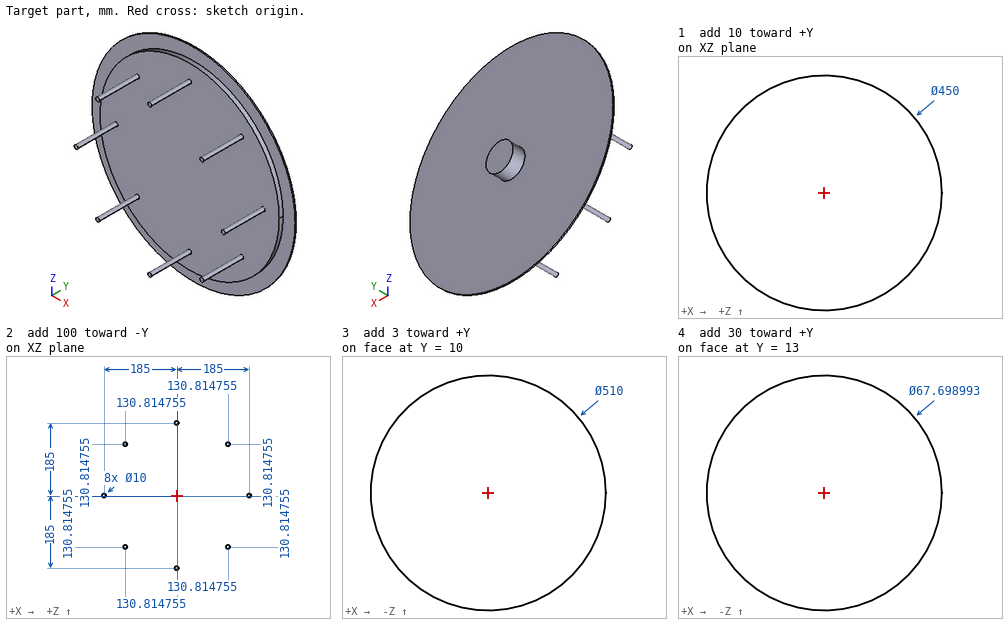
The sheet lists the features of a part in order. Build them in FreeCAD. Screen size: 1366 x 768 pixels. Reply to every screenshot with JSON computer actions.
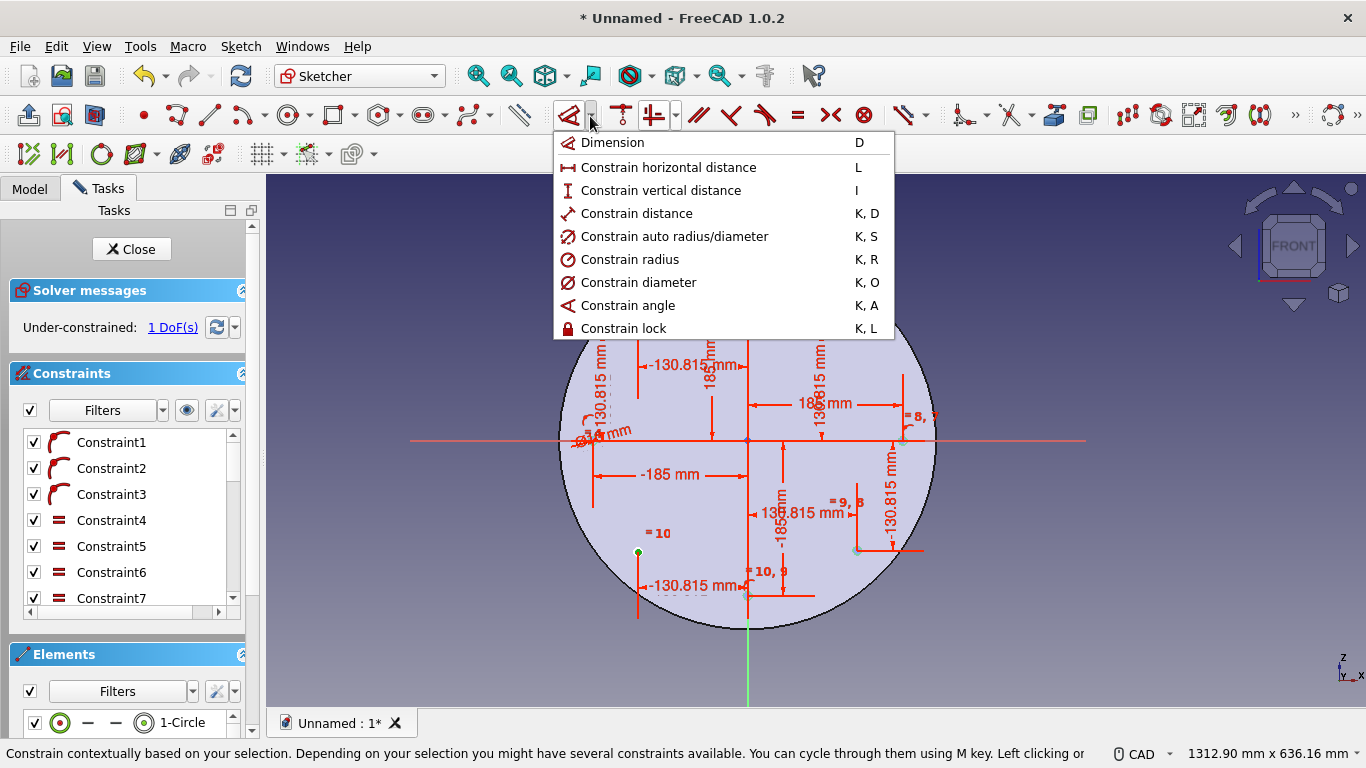
{"action": "left_click", "coordinate": [724, 190]}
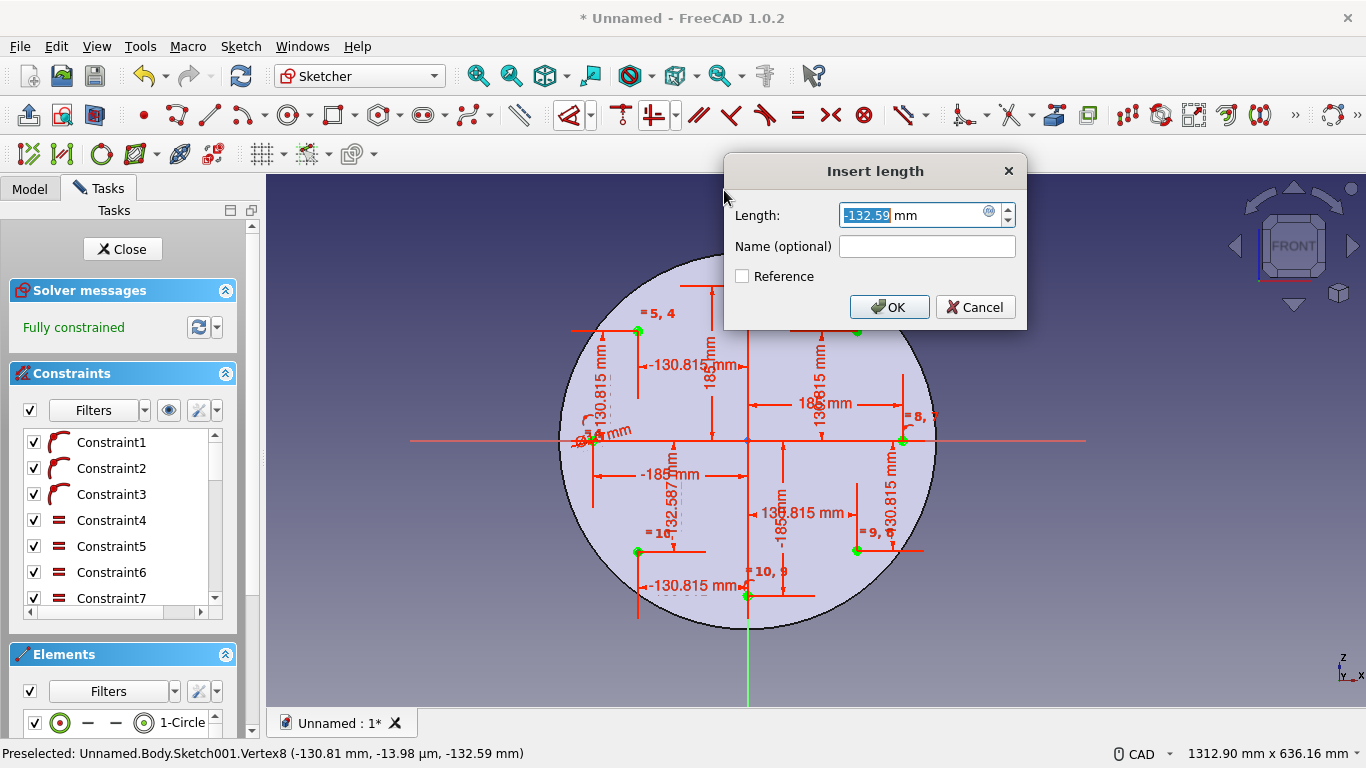
{"action": "type", "text": "-130.814755"}
{"action": "key", "text": "Return"}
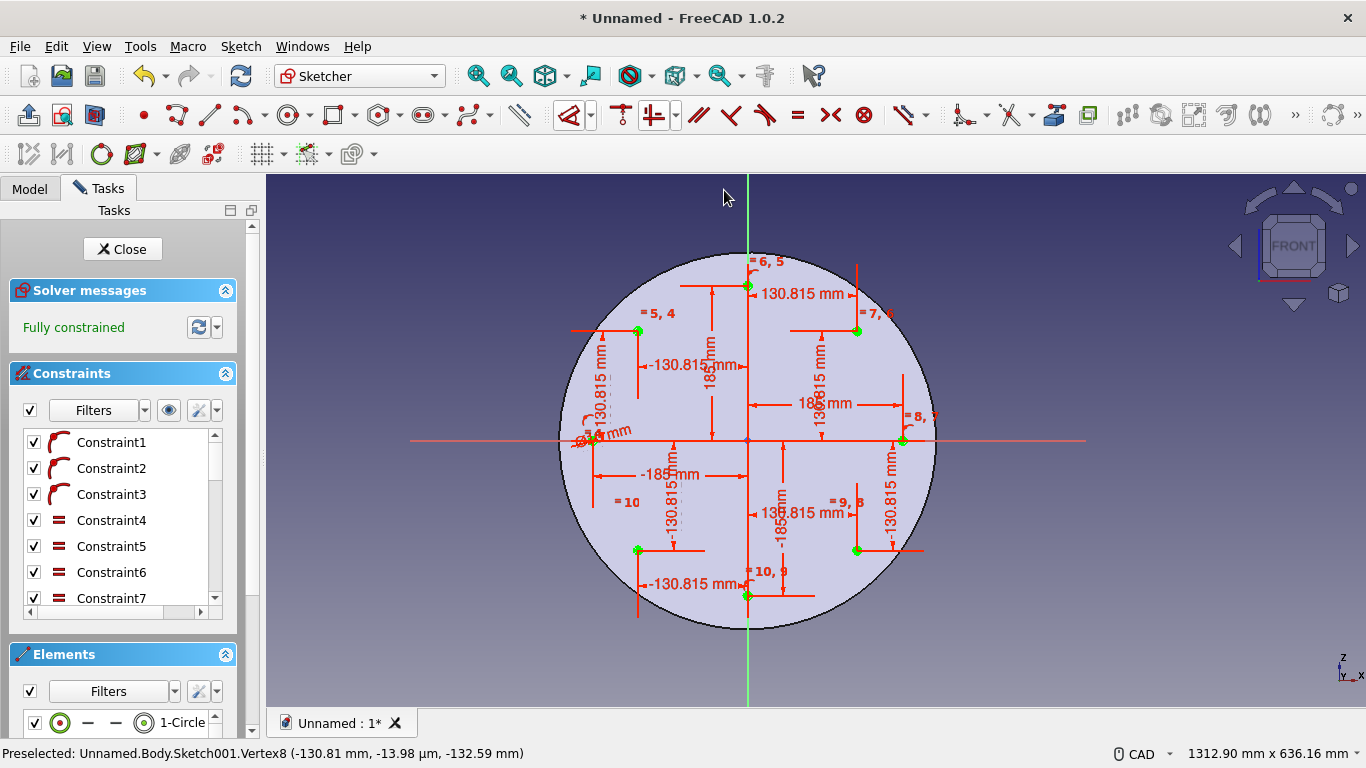
{"action": "left_click", "coordinate": [123, 249]}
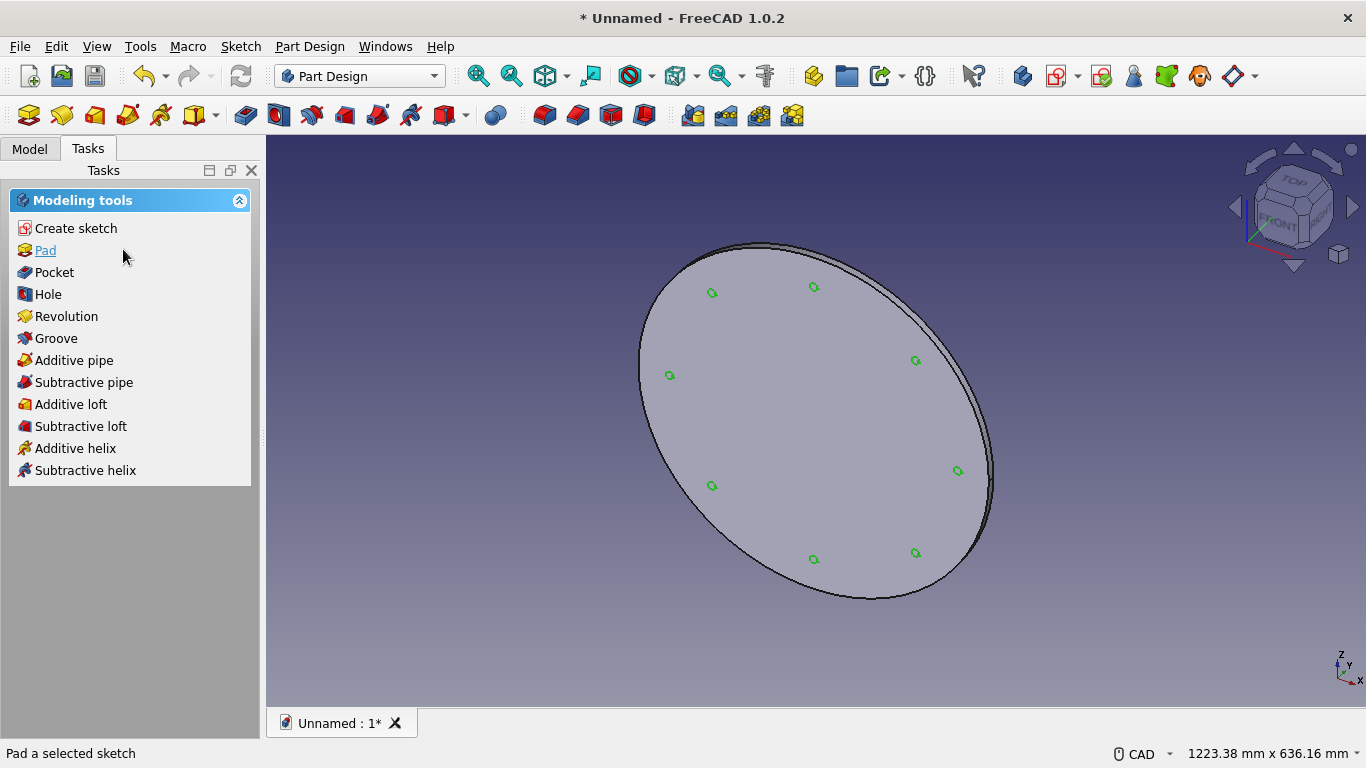
{"action": "left_click", "coordinate": [29, 116]}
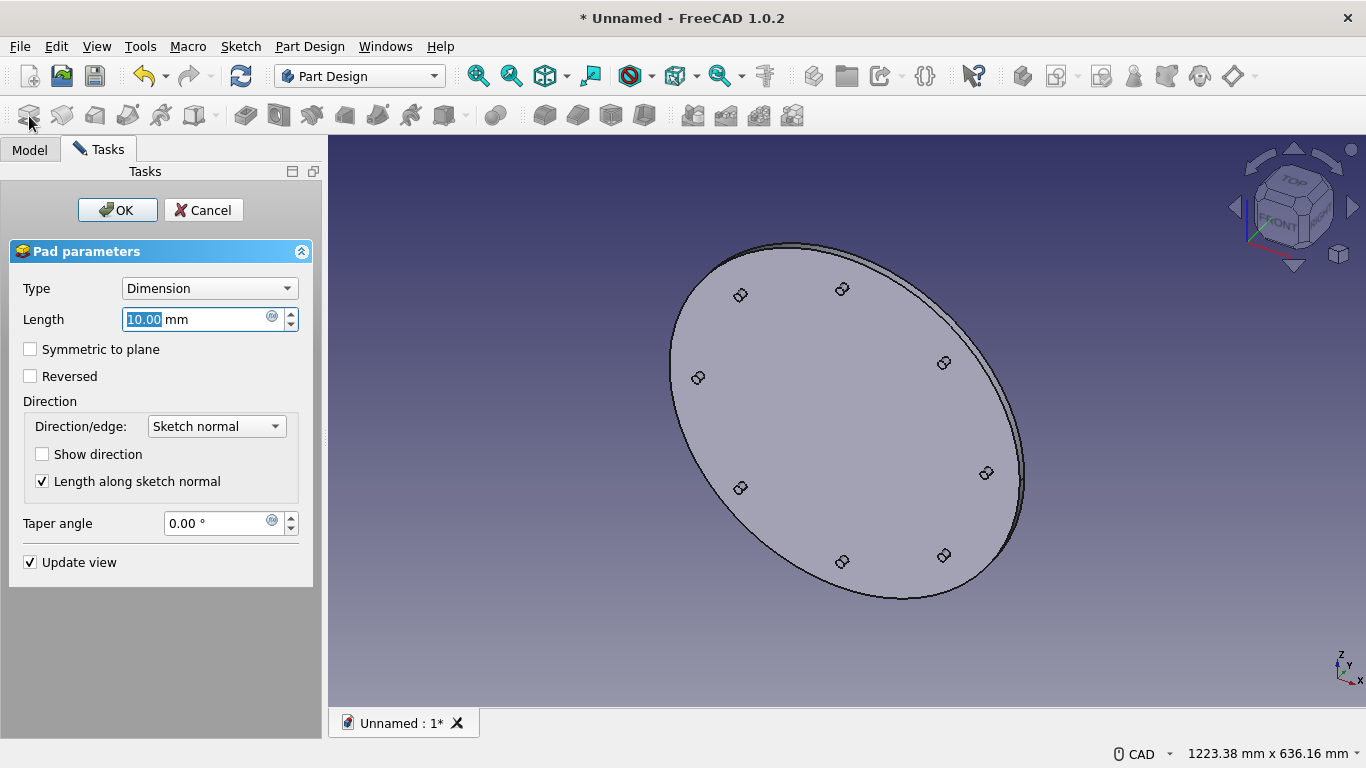
{"action": "type", "text": "100"}
{"action": "key", "text": "Tab"}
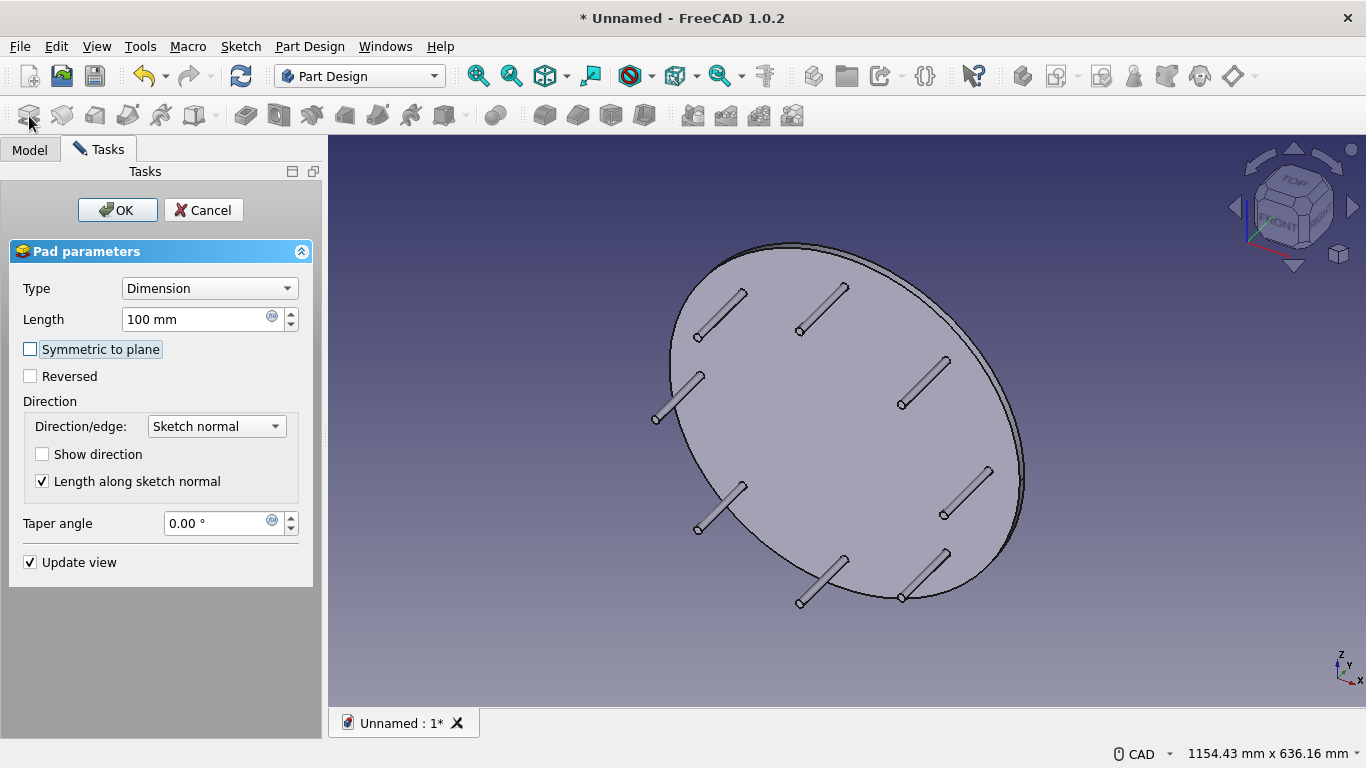
{"action": "left_click", "coordinate": [118, 210]}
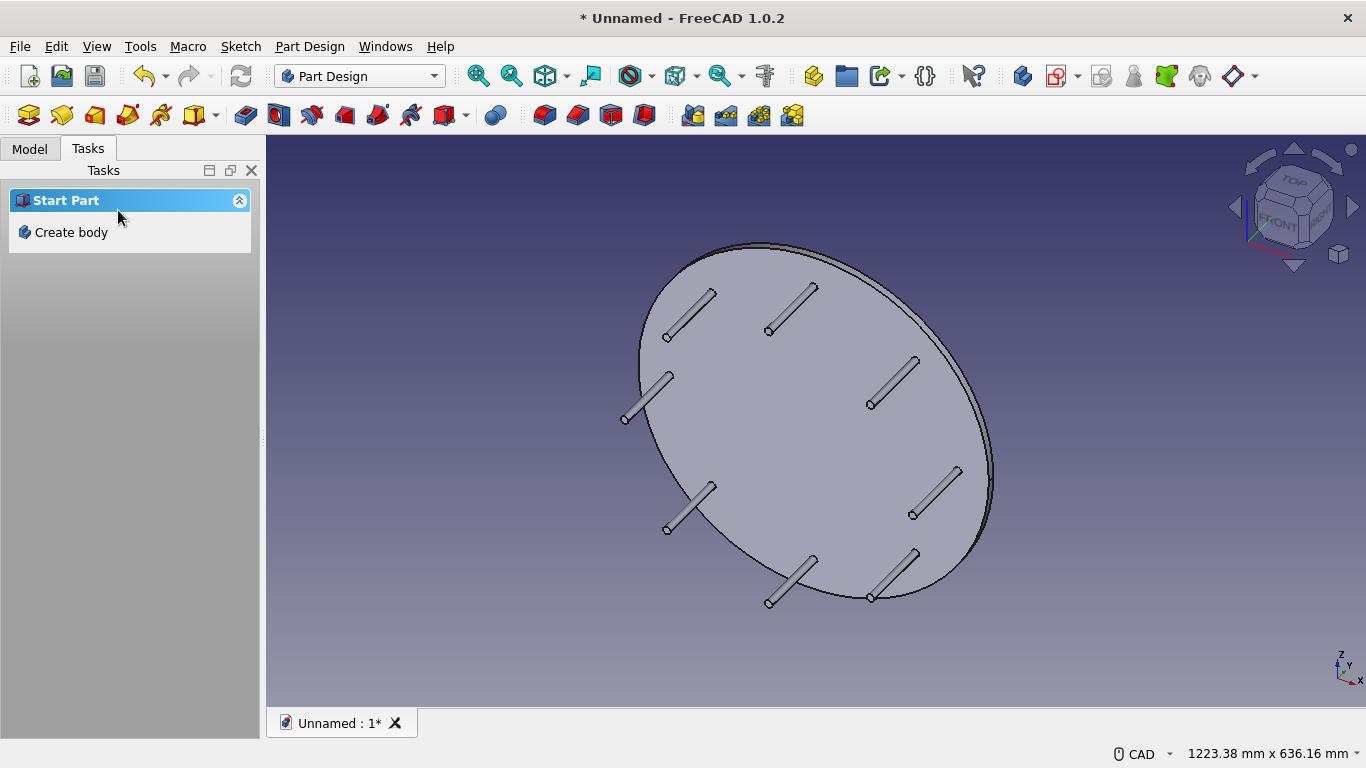
{"action": "key", "text": "4"}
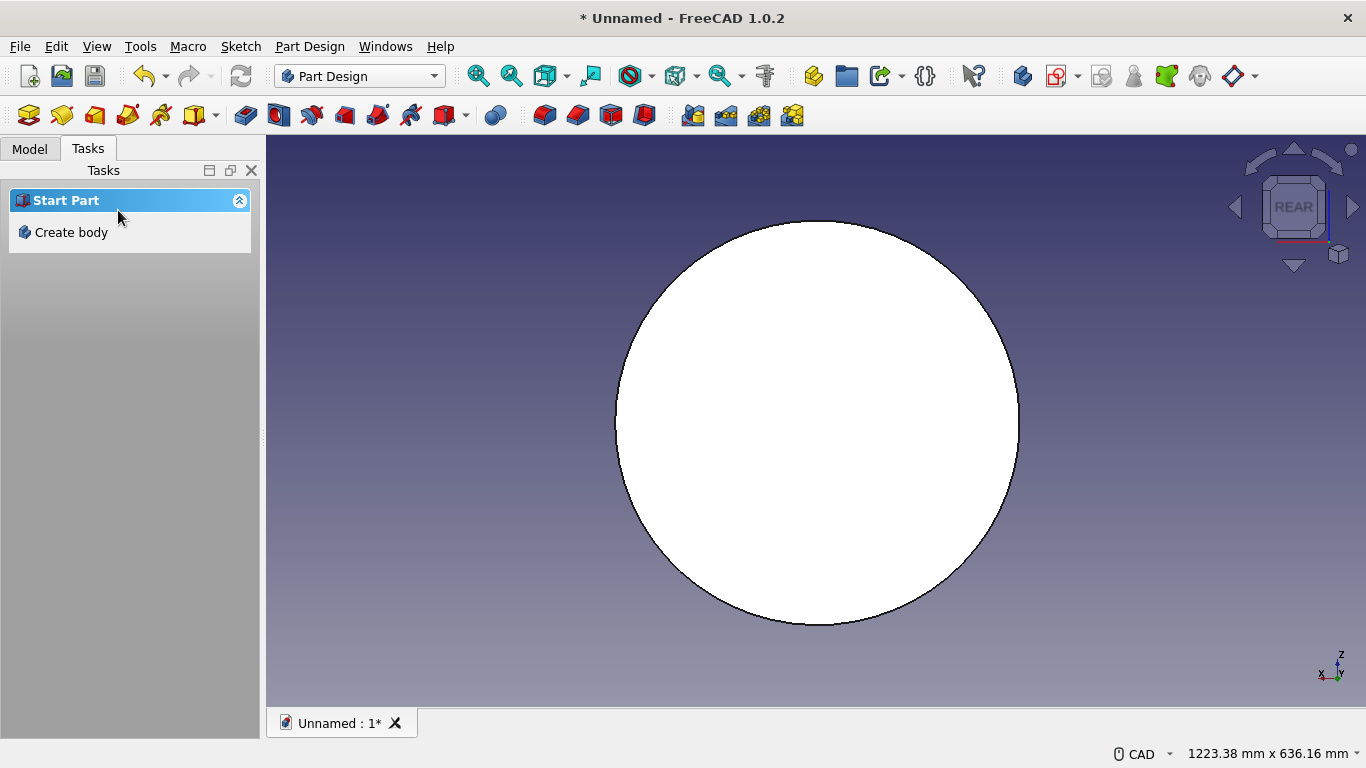
{"action": "left_click", "coordinate": [817, 422]}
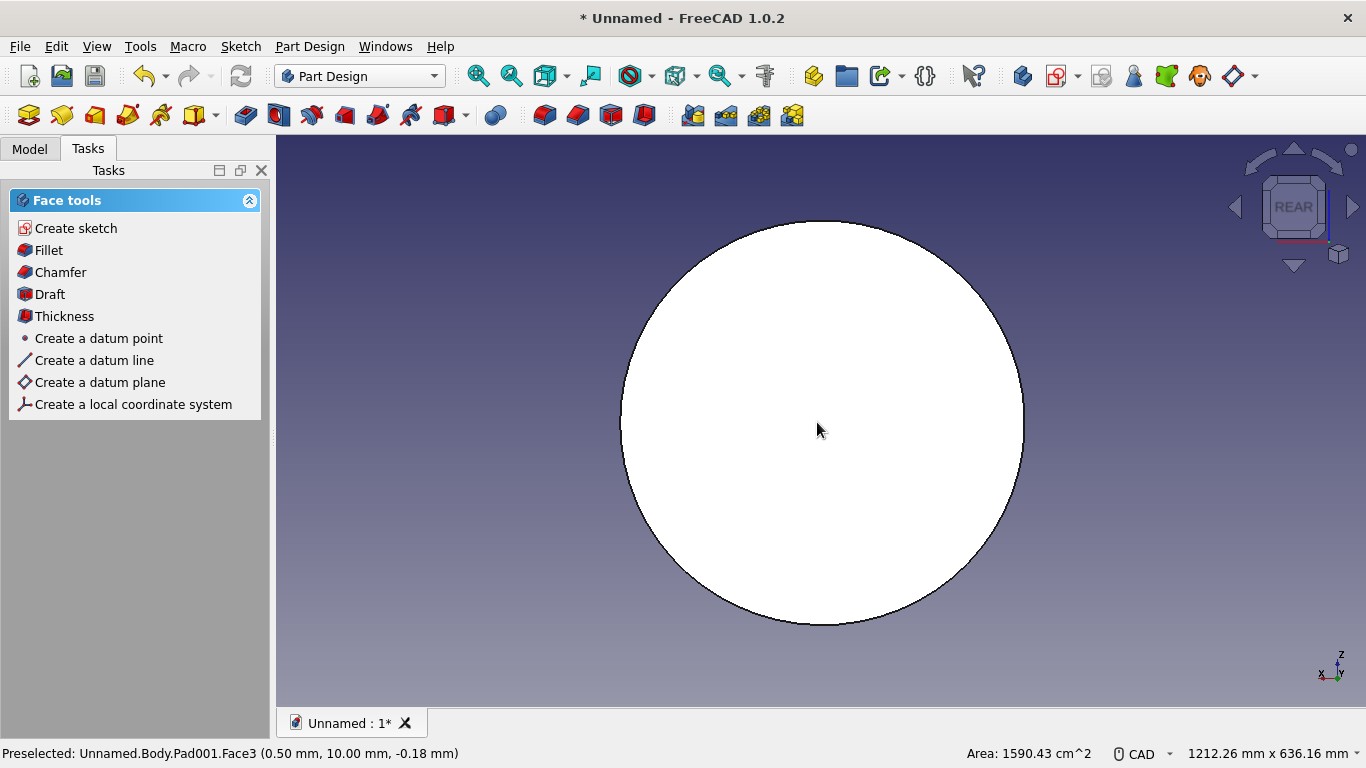
{"action": "left_click", "coordinate": [1056, 76]}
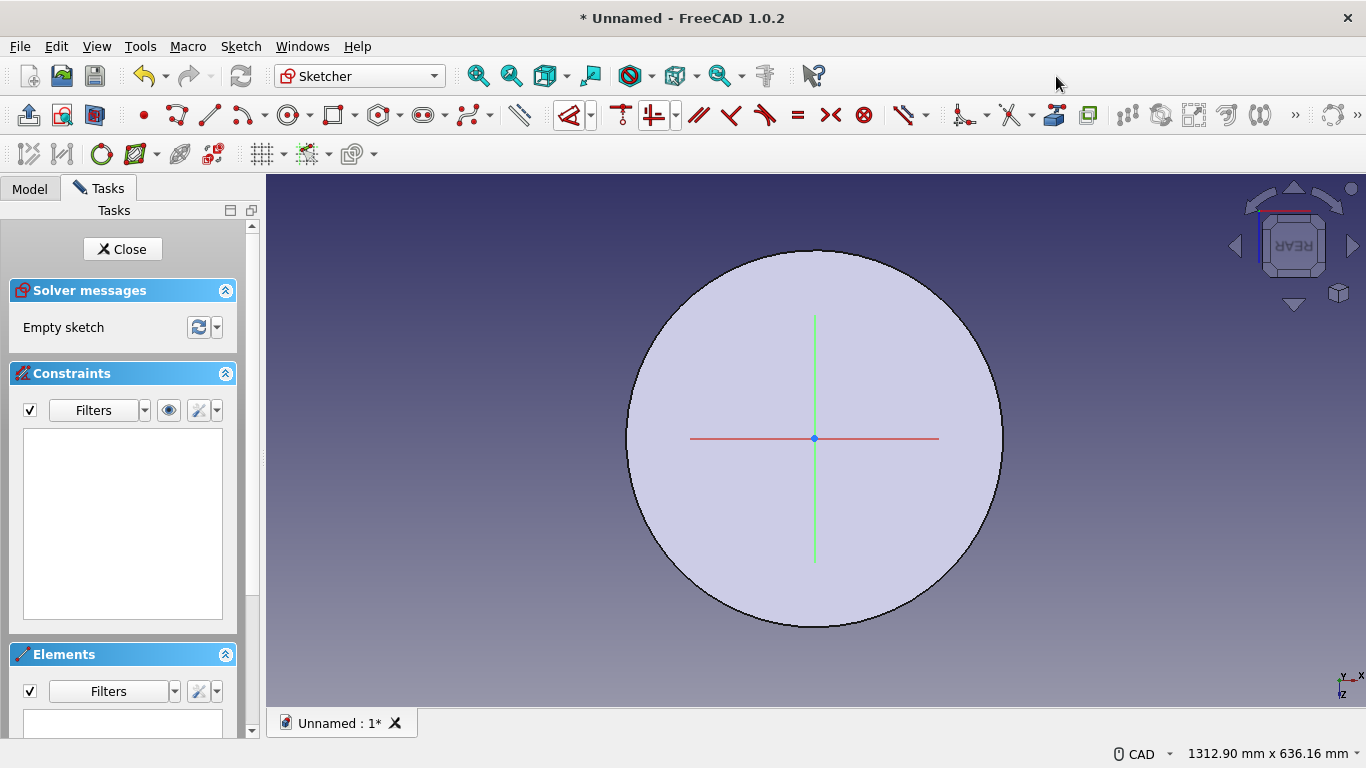
{"action": "scroll", "coordinate": [444, 448], "scroll_direction": "down", "scroll_amount": 1}